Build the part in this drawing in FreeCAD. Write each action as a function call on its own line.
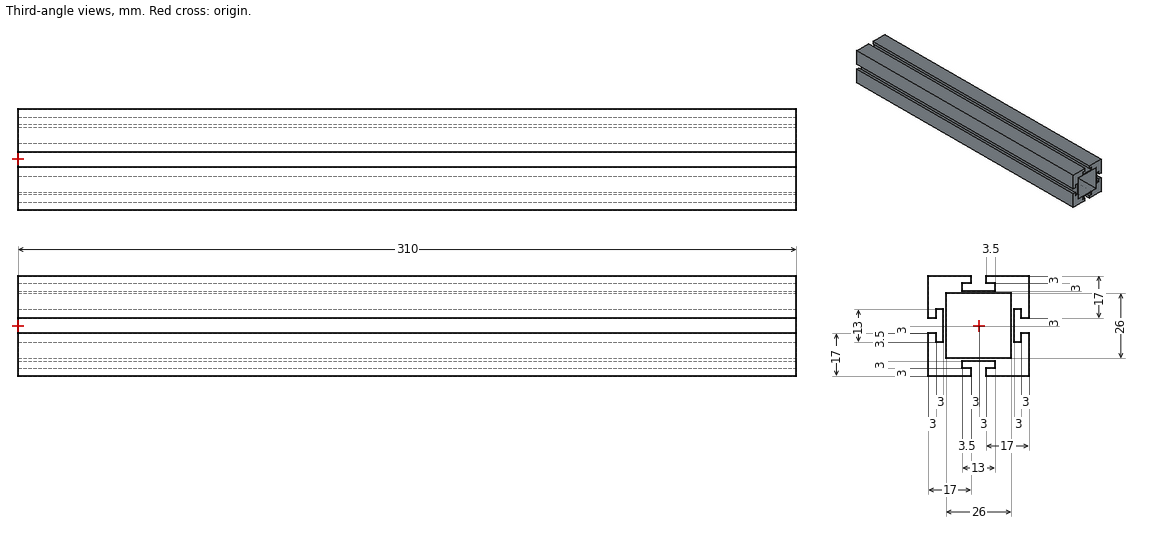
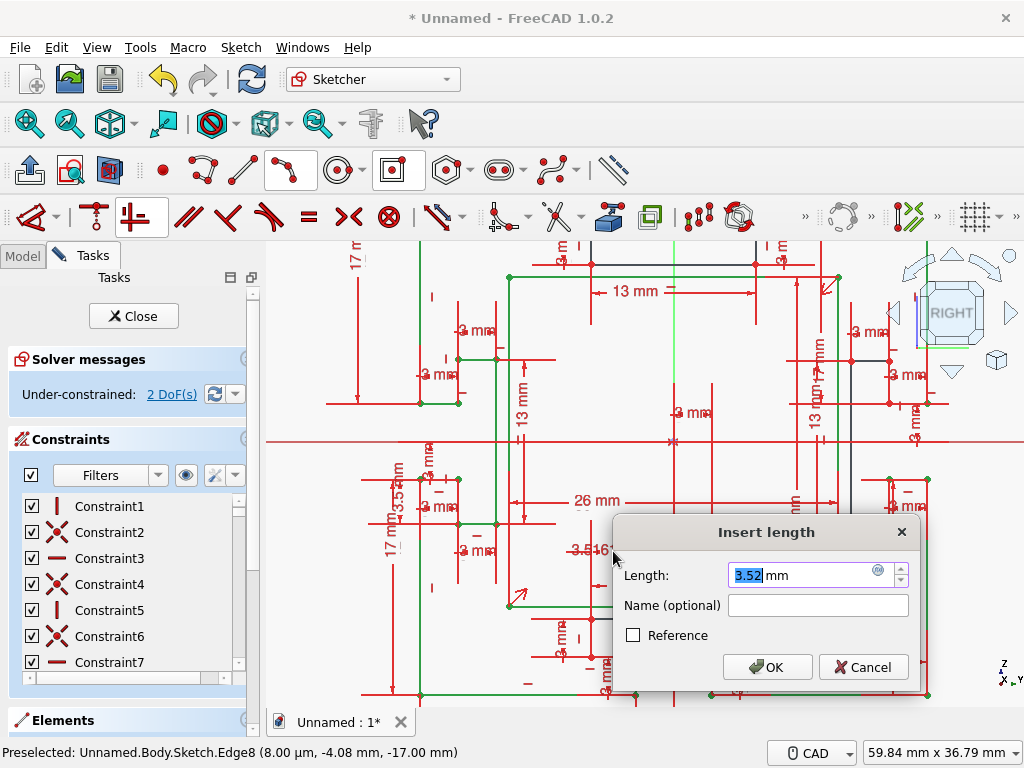
text(3.5)
key(Return)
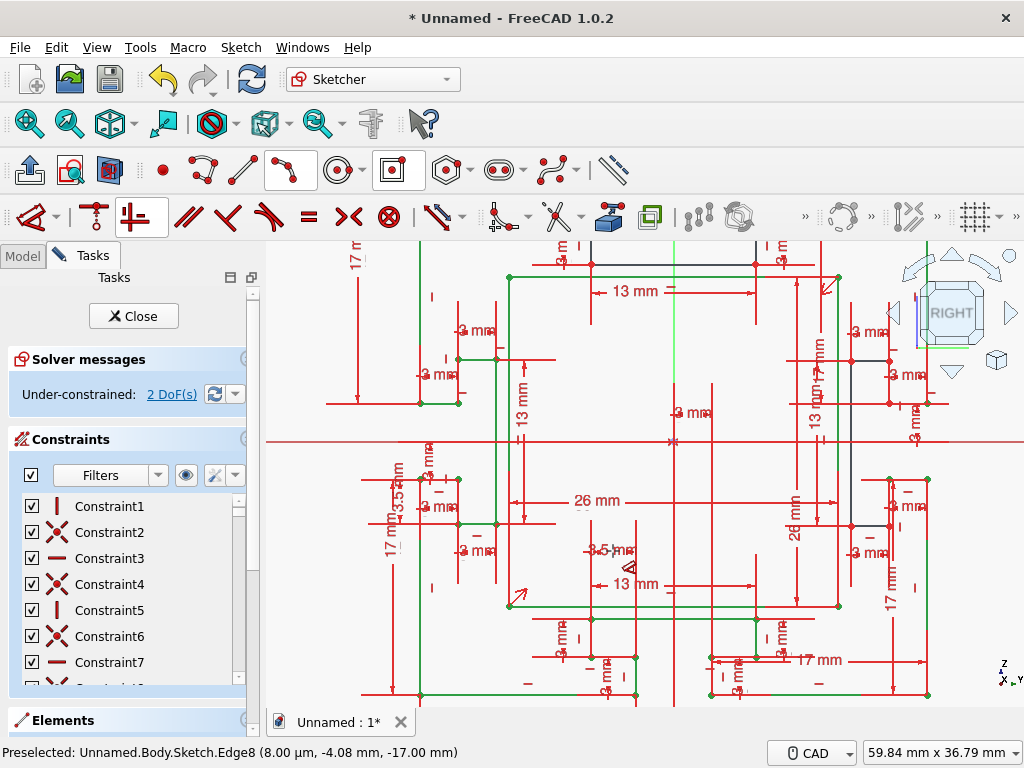
scroll(458, 513, down, 3)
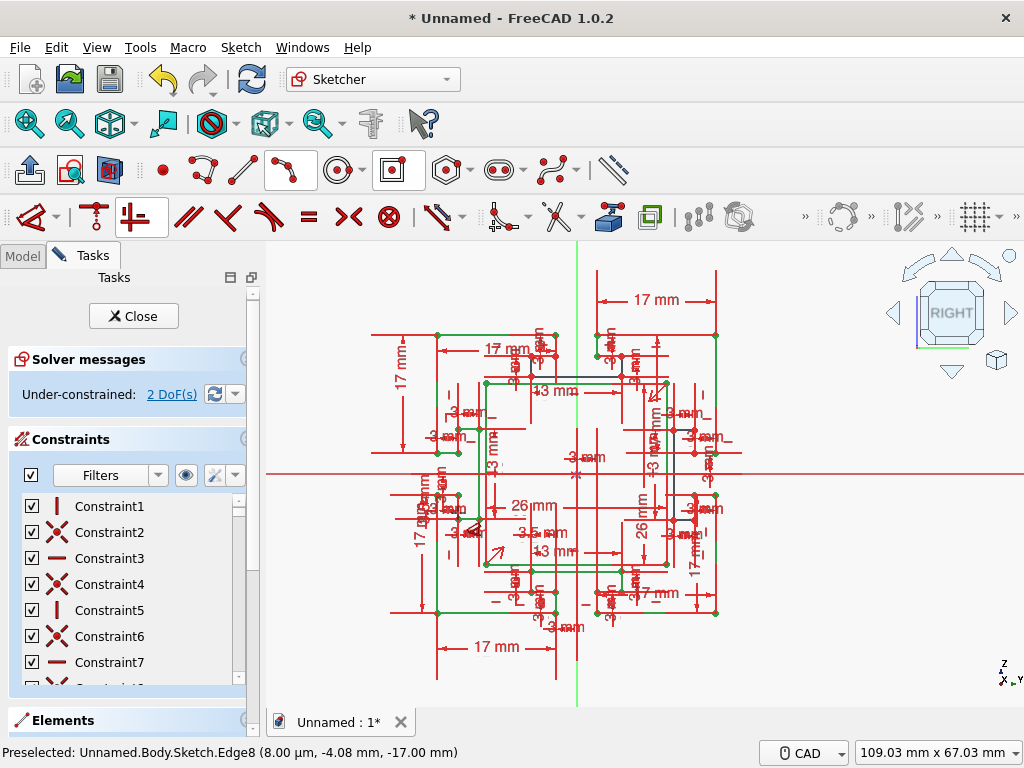
scroll(695, 503, up, 3)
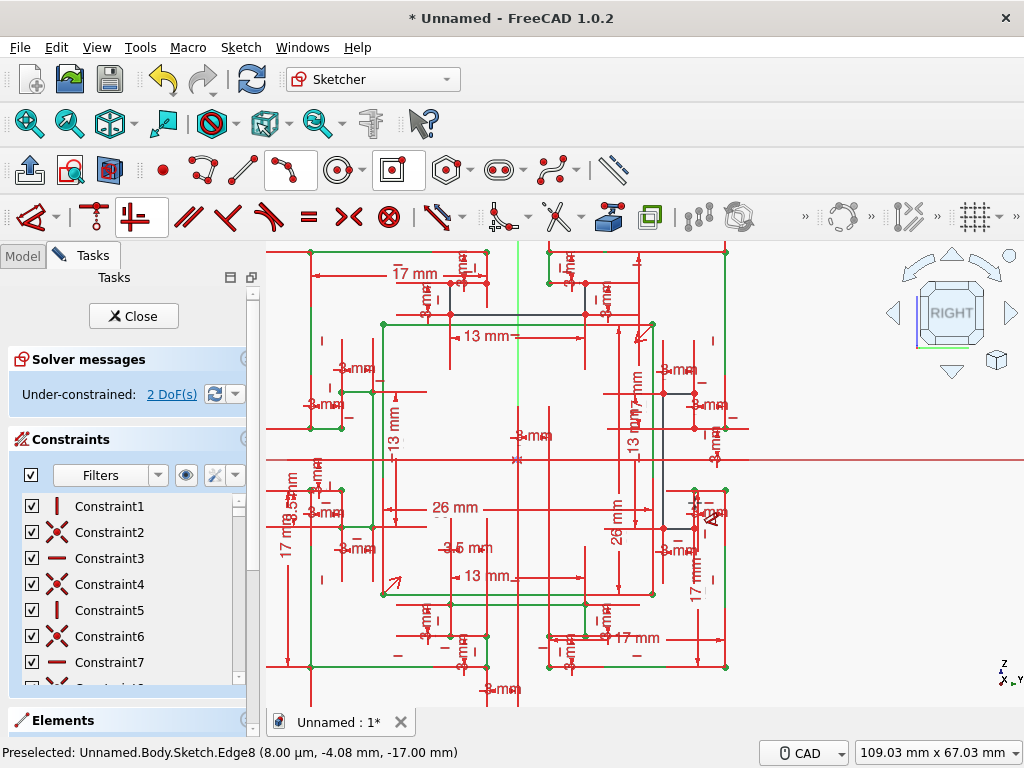
click(694, 502)
click(752, 495)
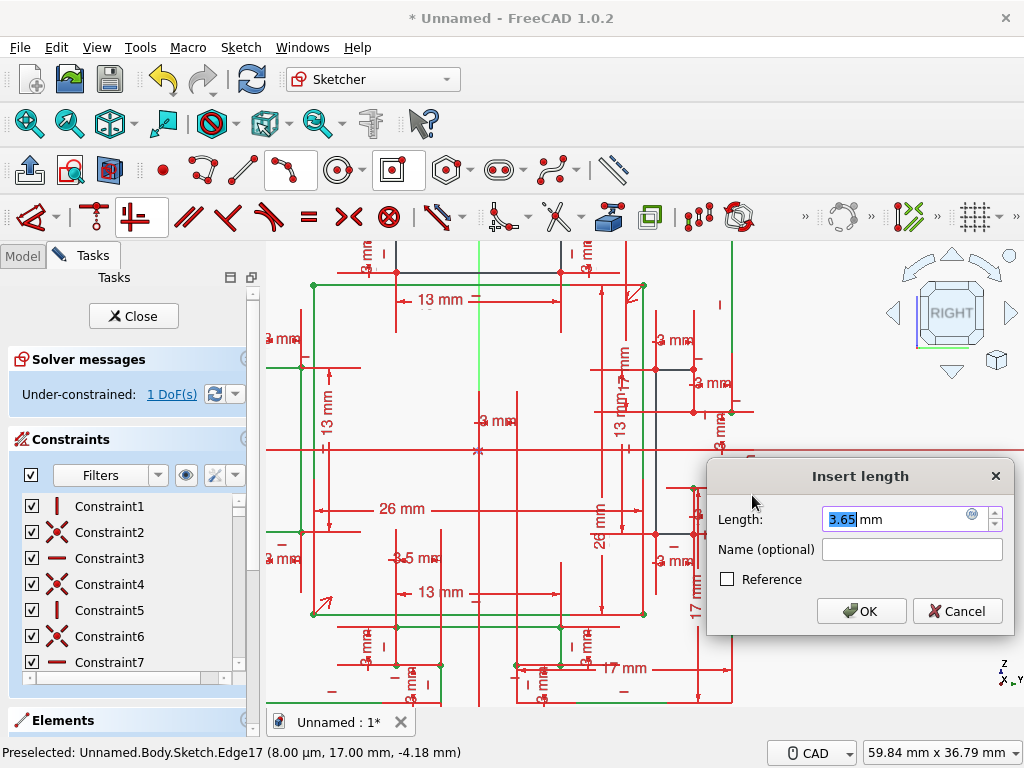
text(3.5)
key(Return)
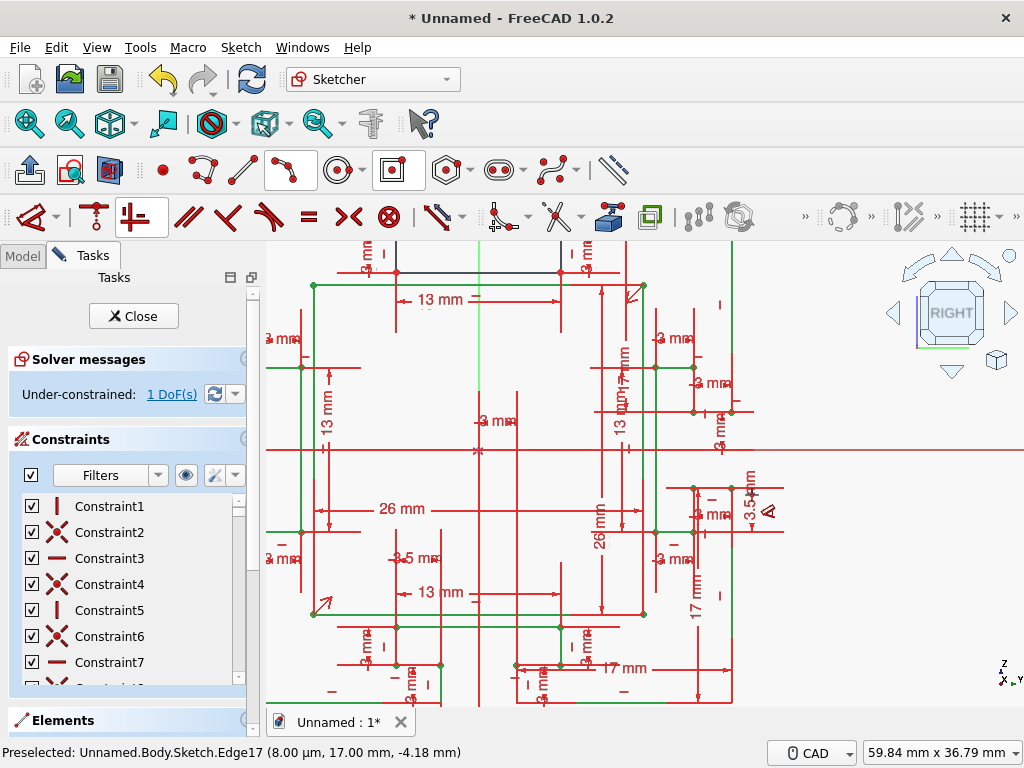
scroll(696, 503, down, 3)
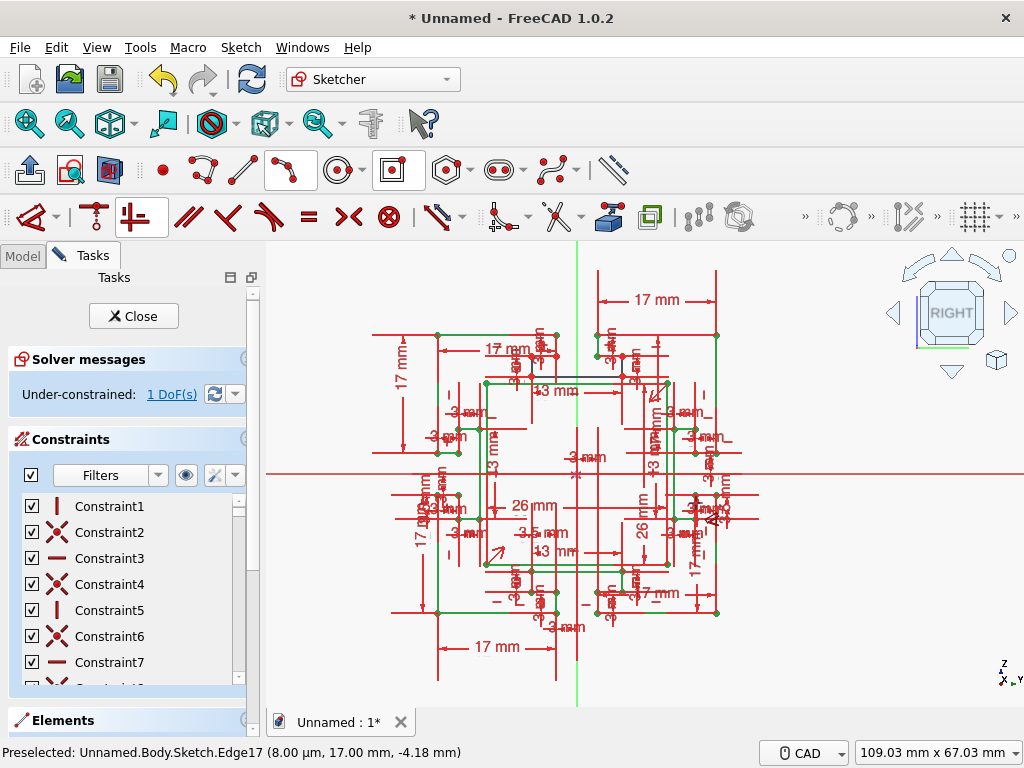
scroll(605, 356, up, 4)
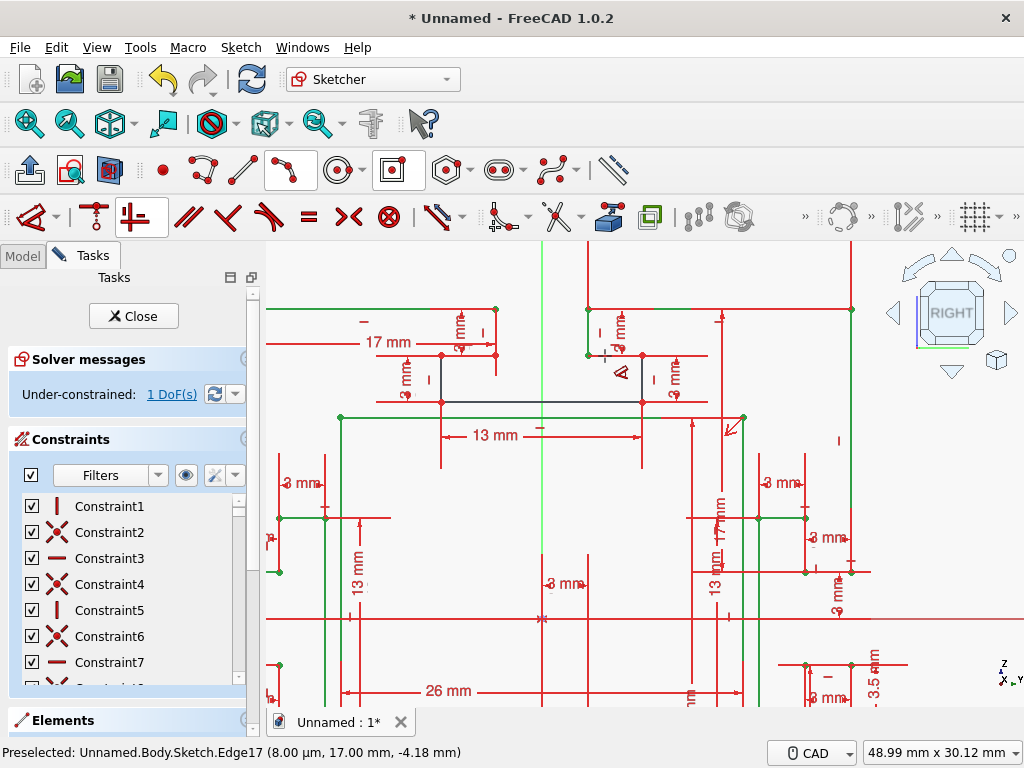
click(605, 356)
click(615, 274)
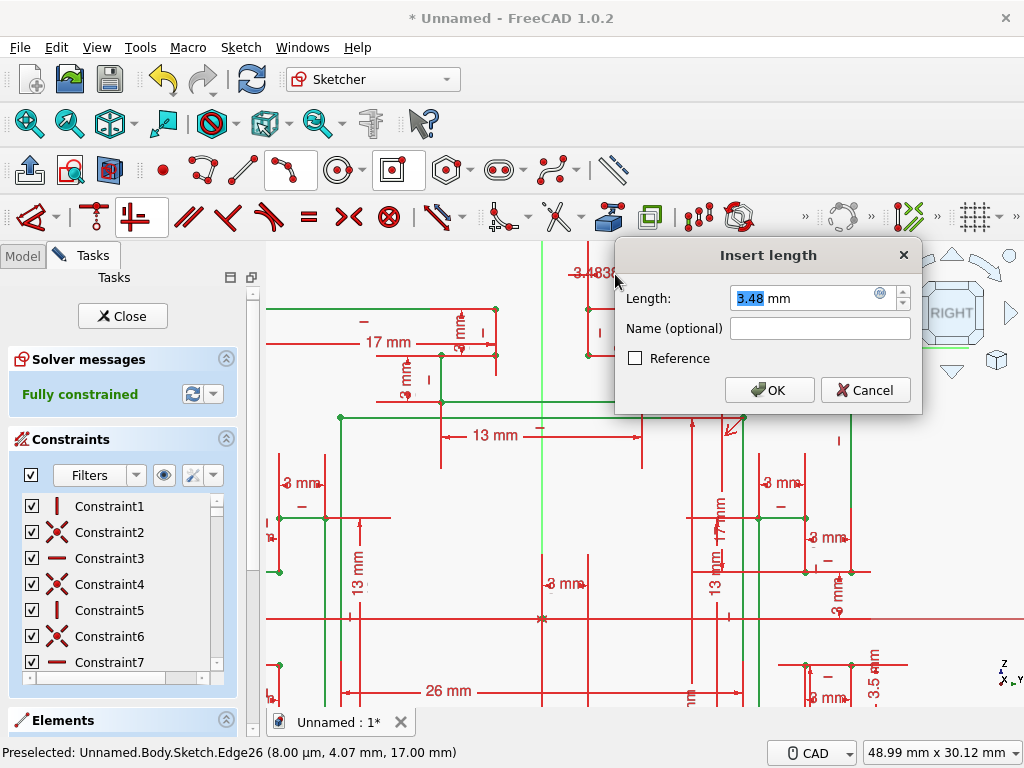
text(3.5)
key(Return)
key(Escape)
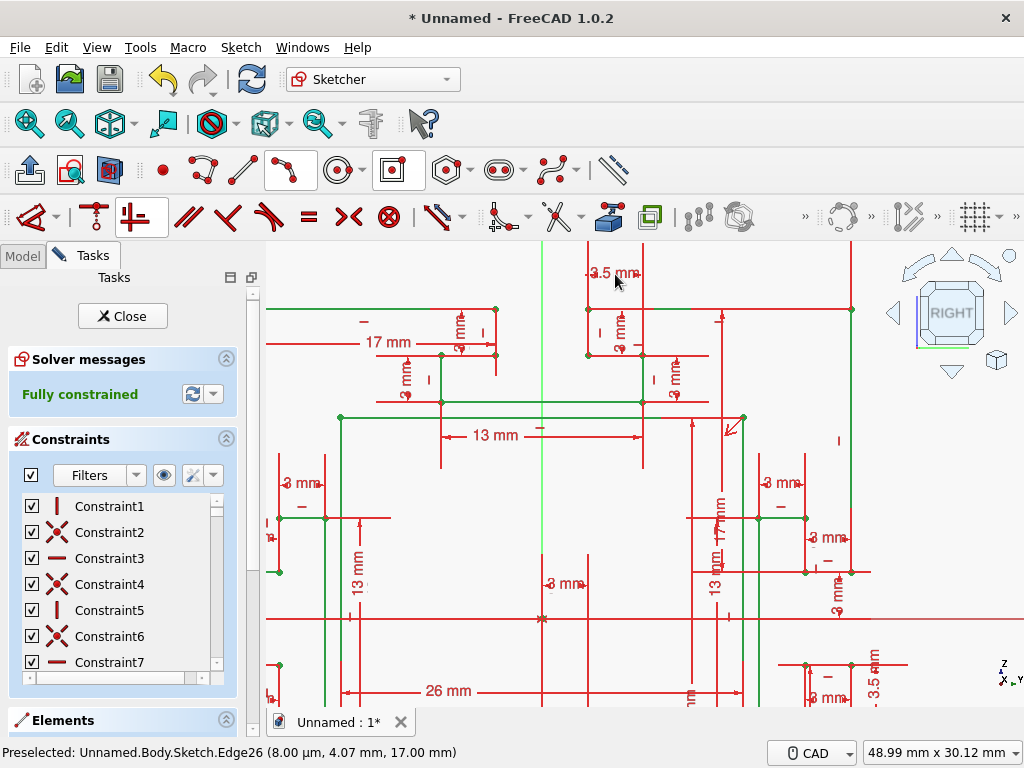
click(123, 316)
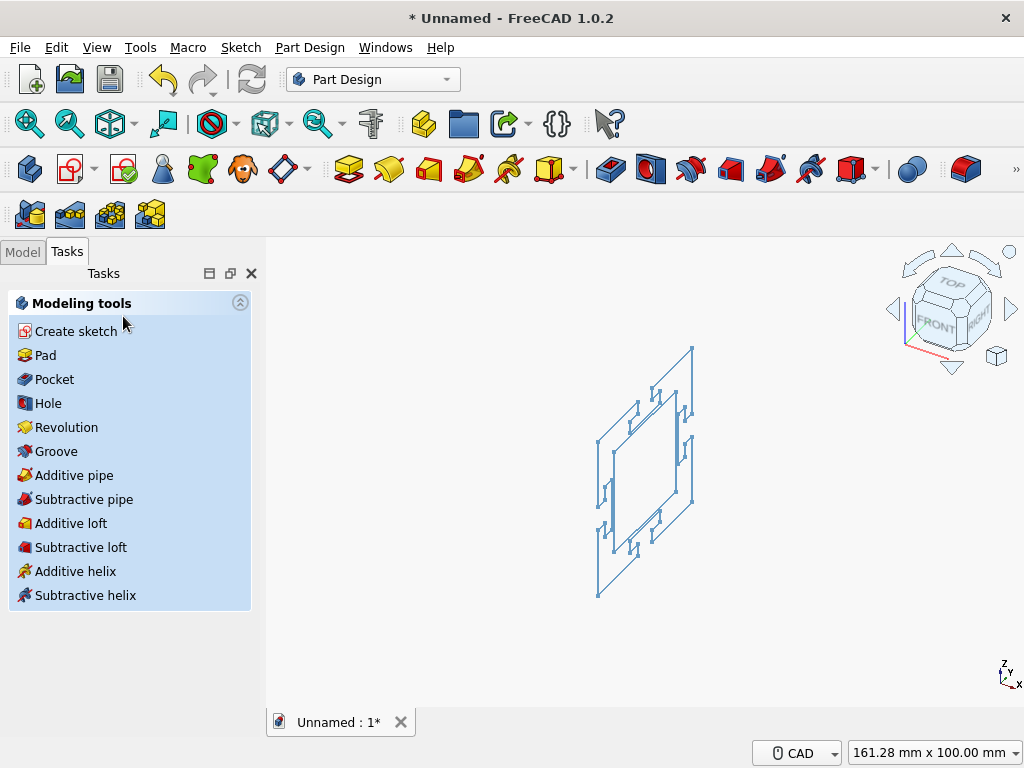
click(350, 170)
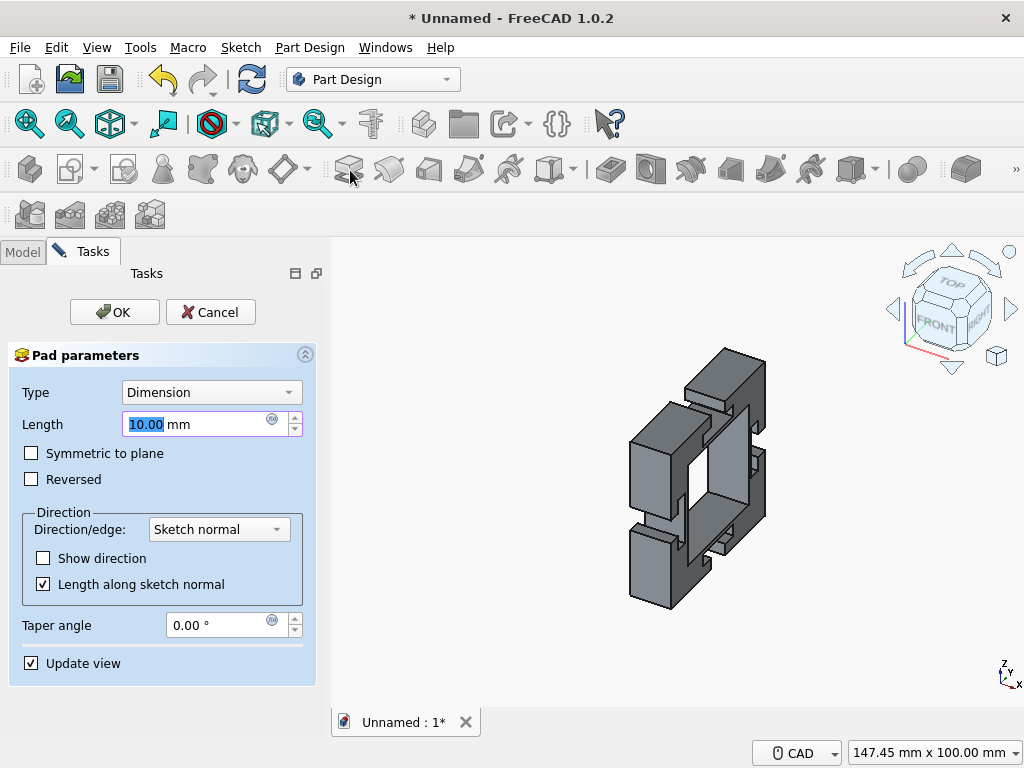
text(310)
key(Tab)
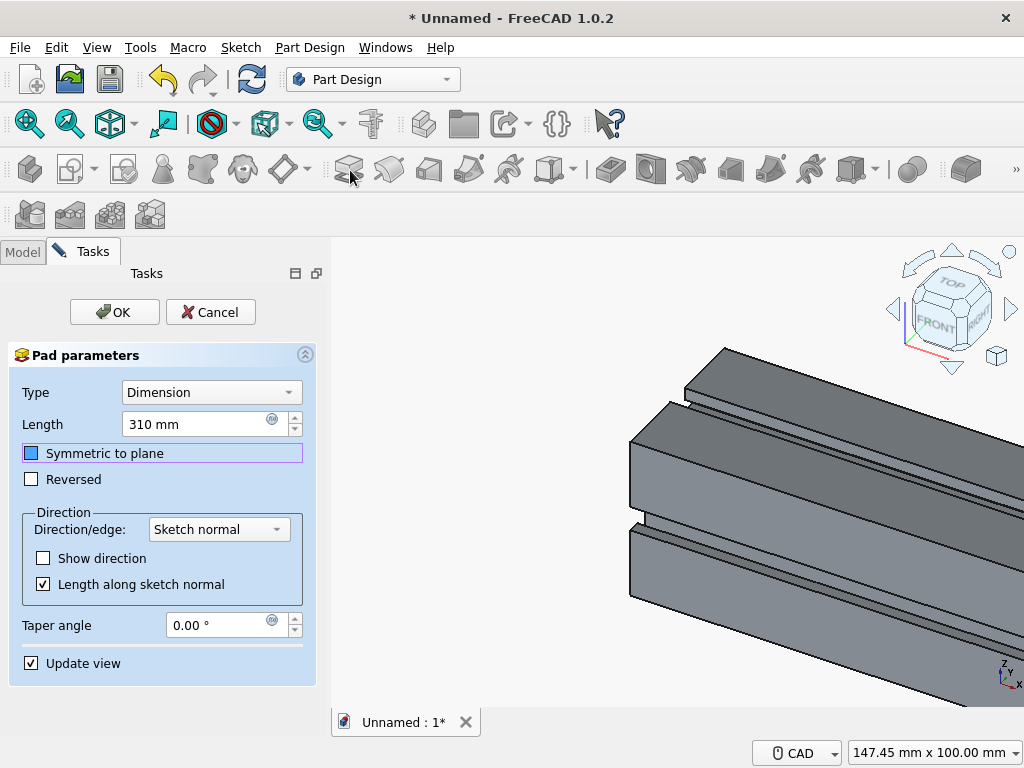
click(115, 312)